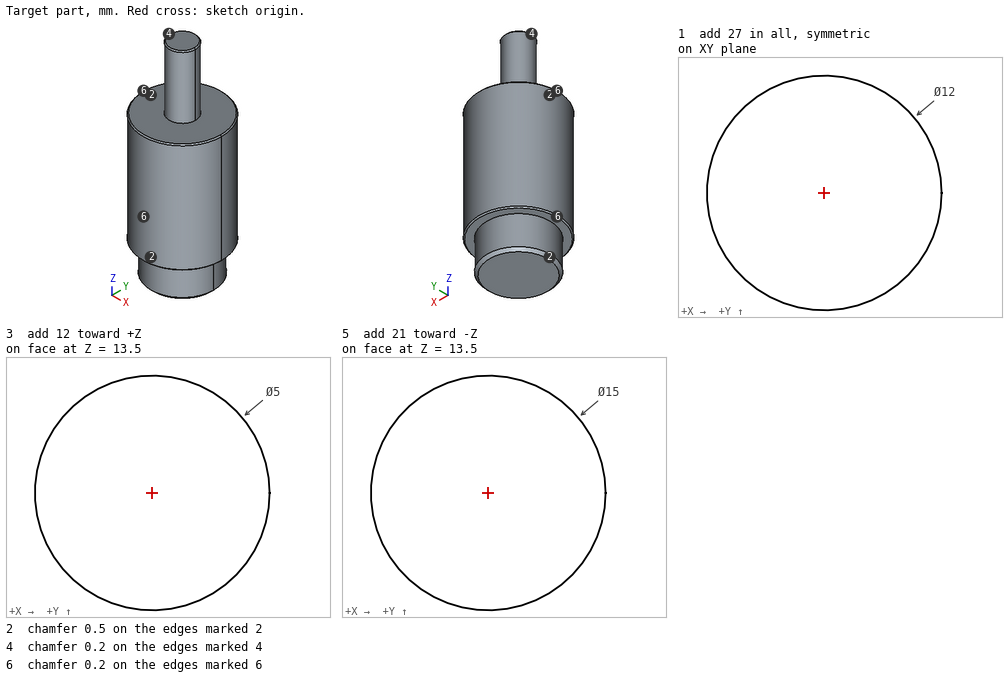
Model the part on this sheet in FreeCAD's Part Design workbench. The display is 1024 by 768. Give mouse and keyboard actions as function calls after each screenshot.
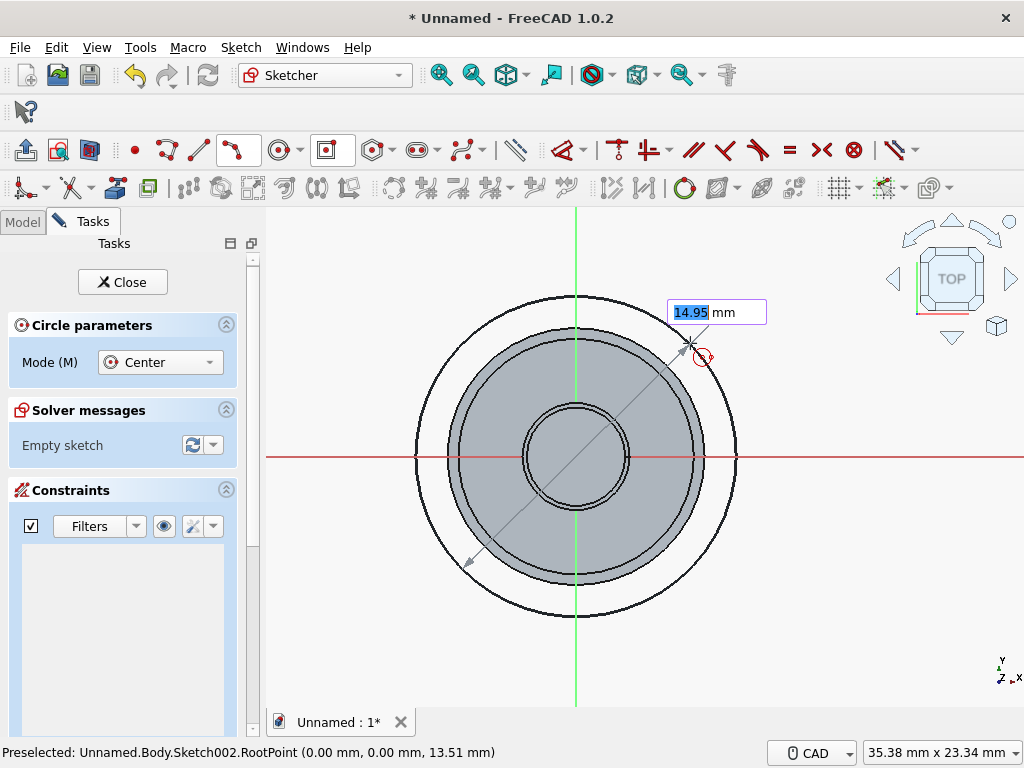
text(15)
key(Return)
key(Escape)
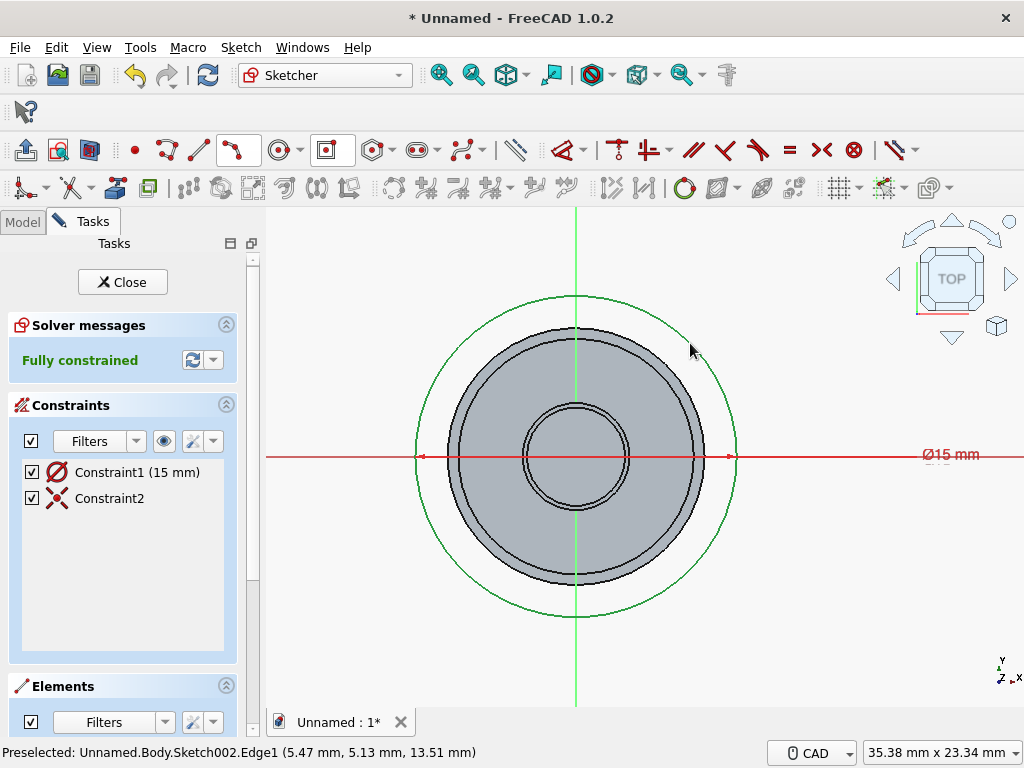
click(123, 282)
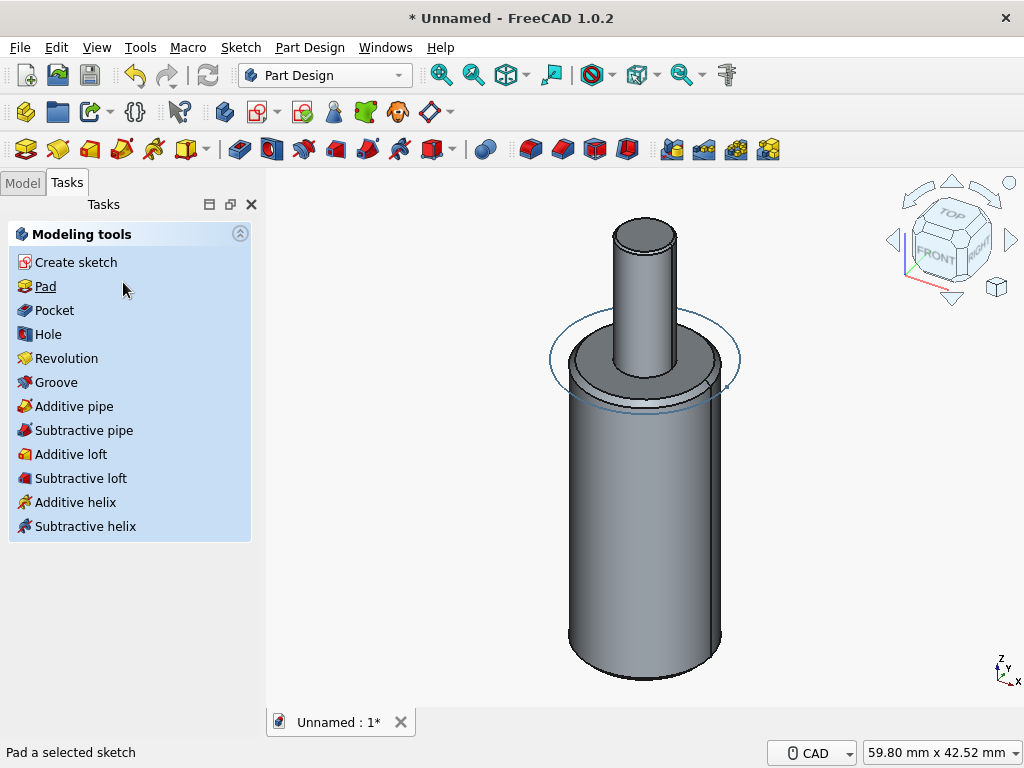
click(26, 150)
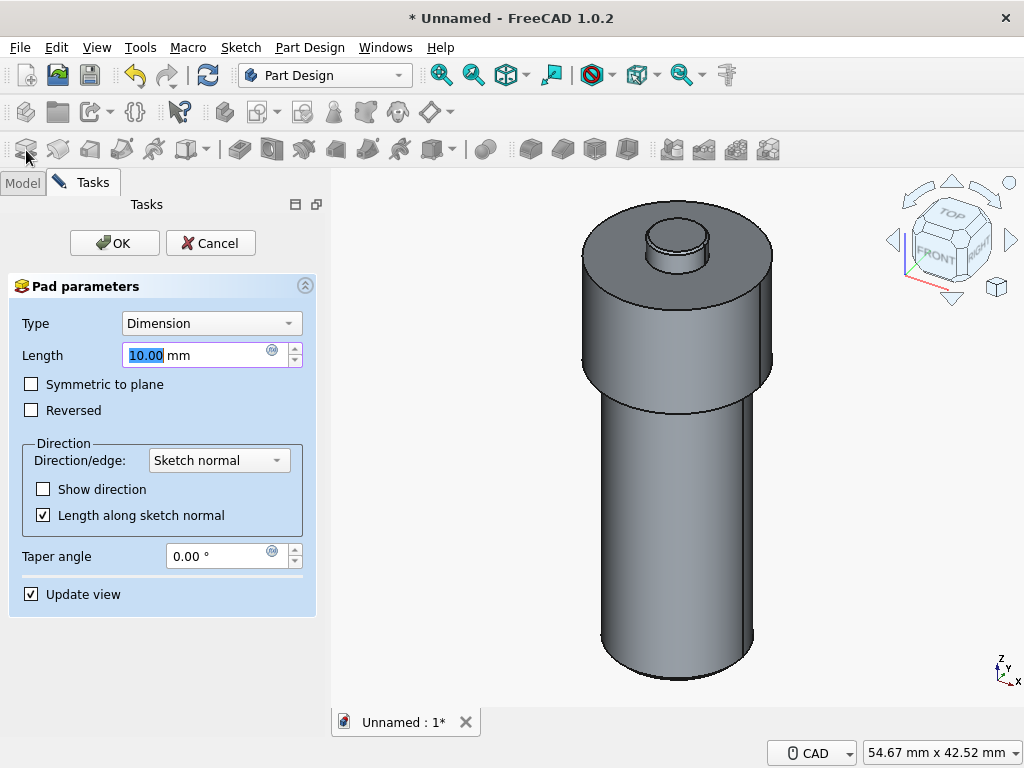
text(21)
key(Tab)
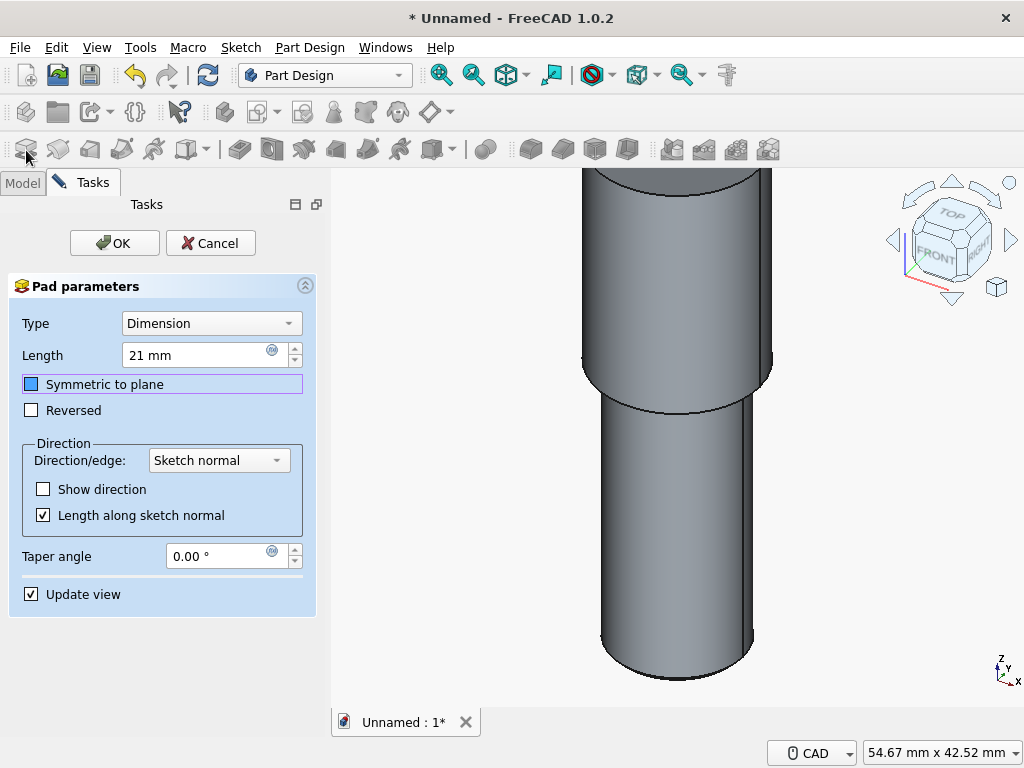
click(30, 410)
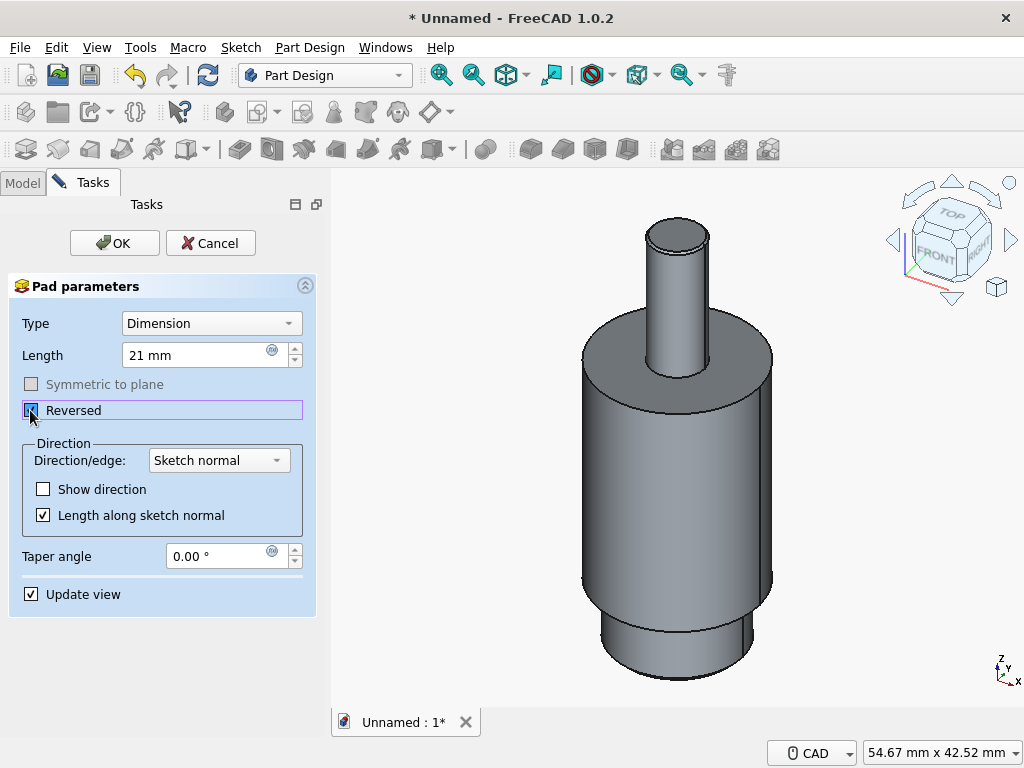
click(115, 243)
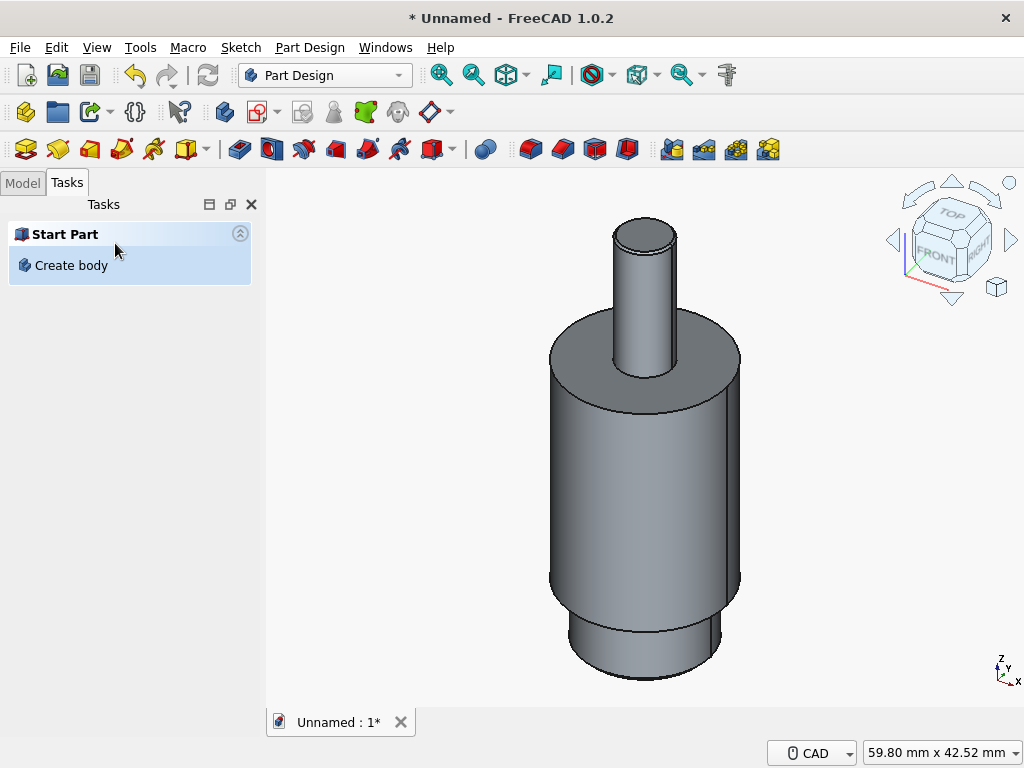
key(v)
key(f)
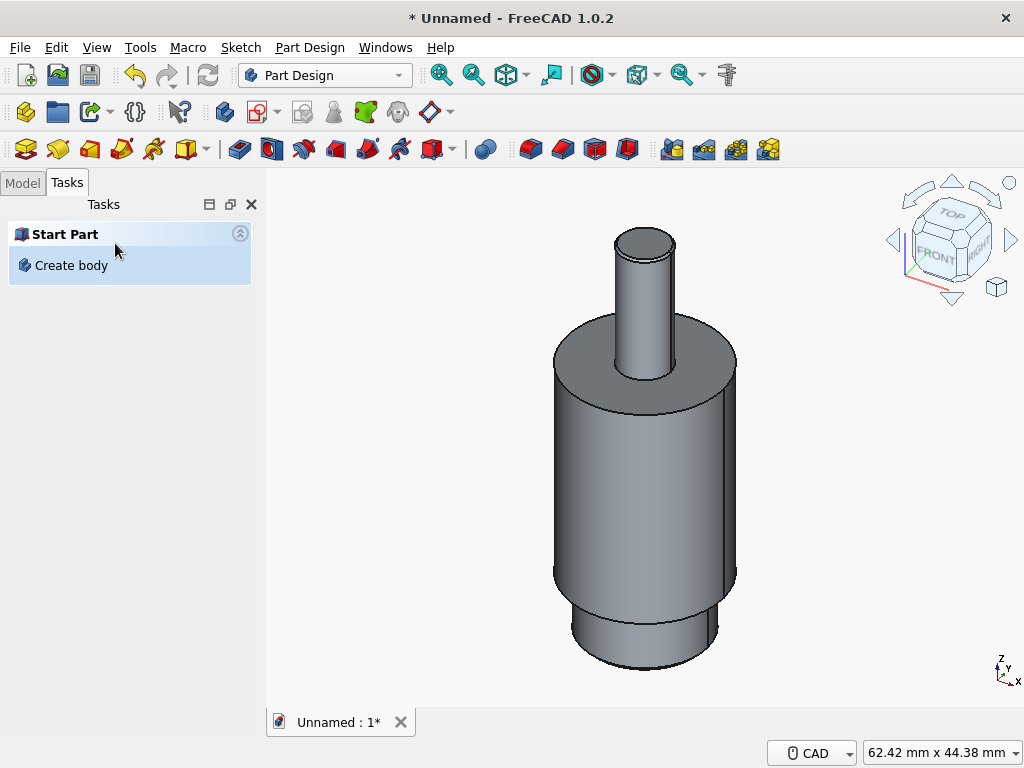
click(554, 367)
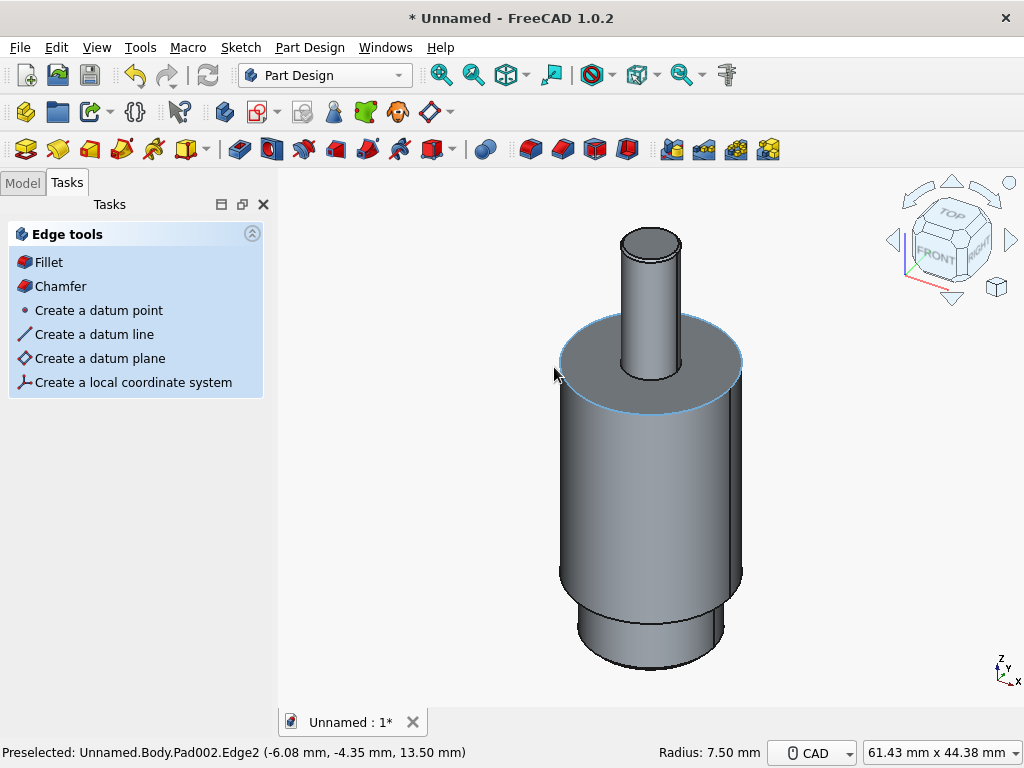
click(583, 606, ctrl)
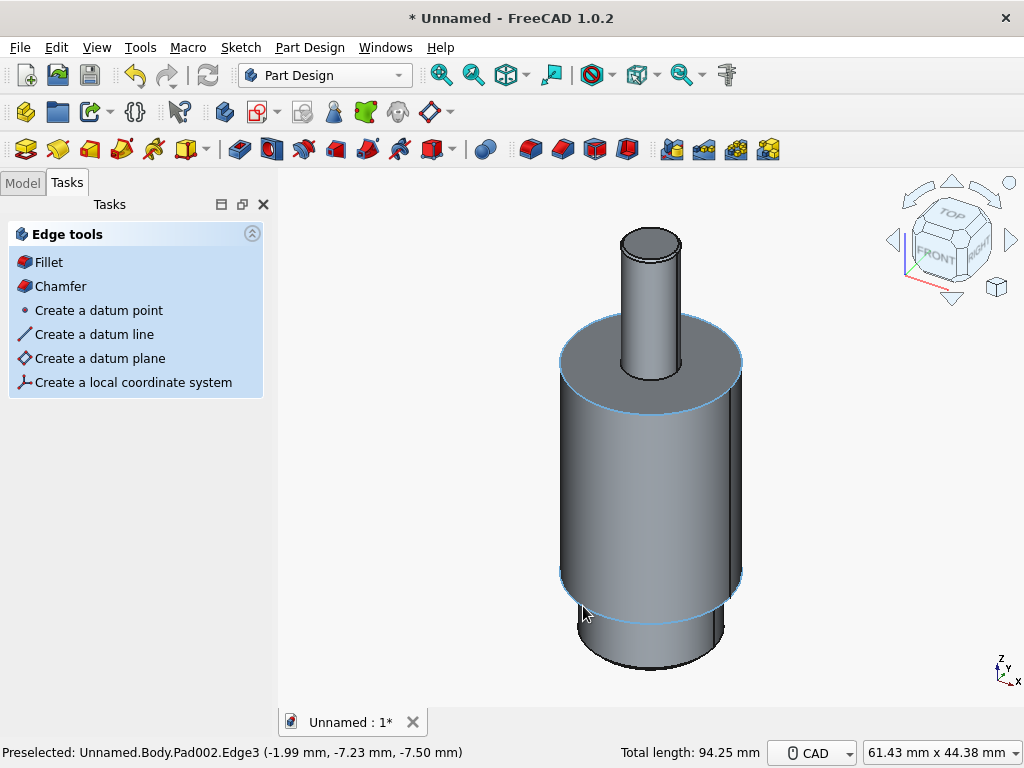
click(564, 150)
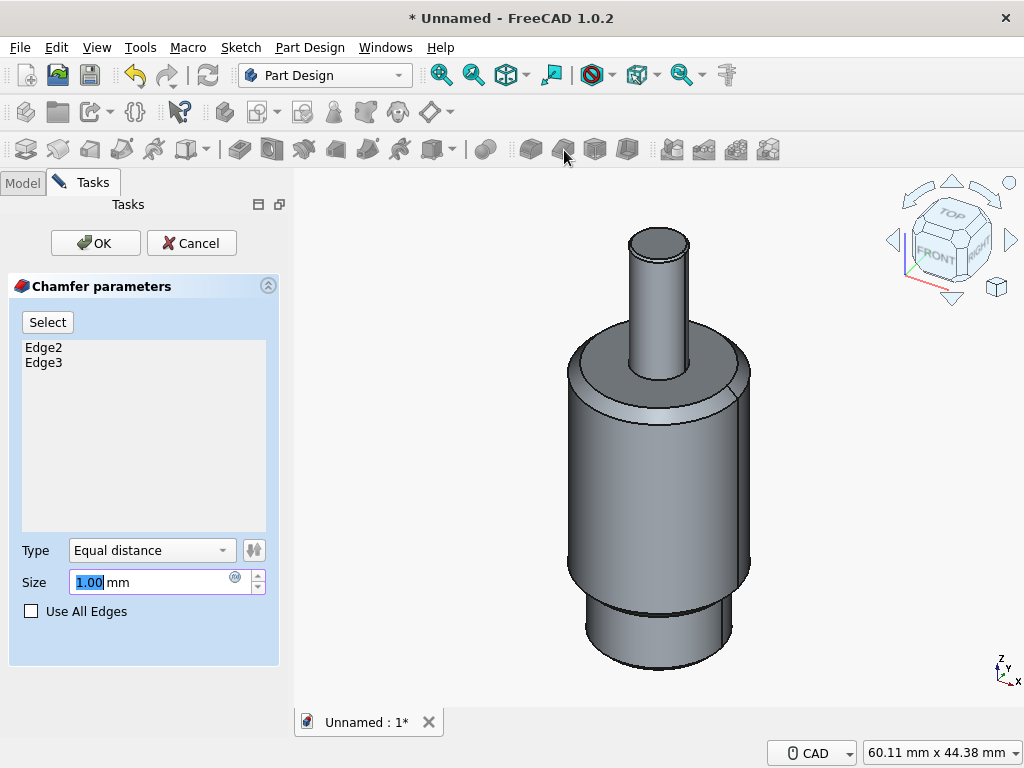
text(0.2)
key(Tab)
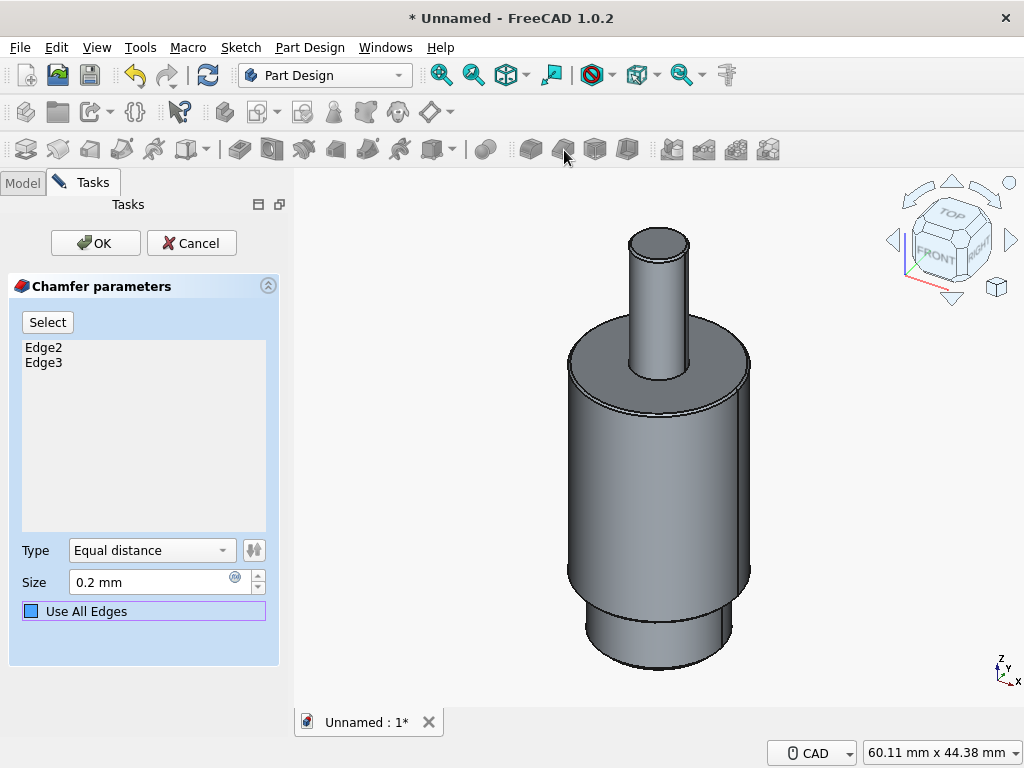
click(96, 243)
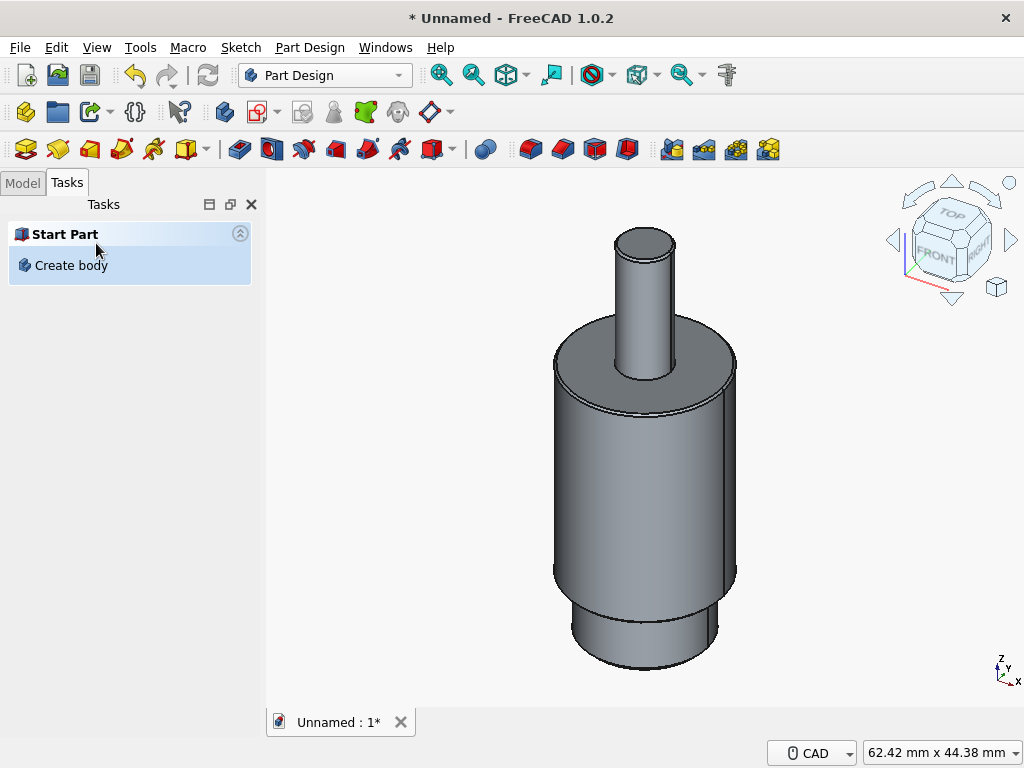
key(0)